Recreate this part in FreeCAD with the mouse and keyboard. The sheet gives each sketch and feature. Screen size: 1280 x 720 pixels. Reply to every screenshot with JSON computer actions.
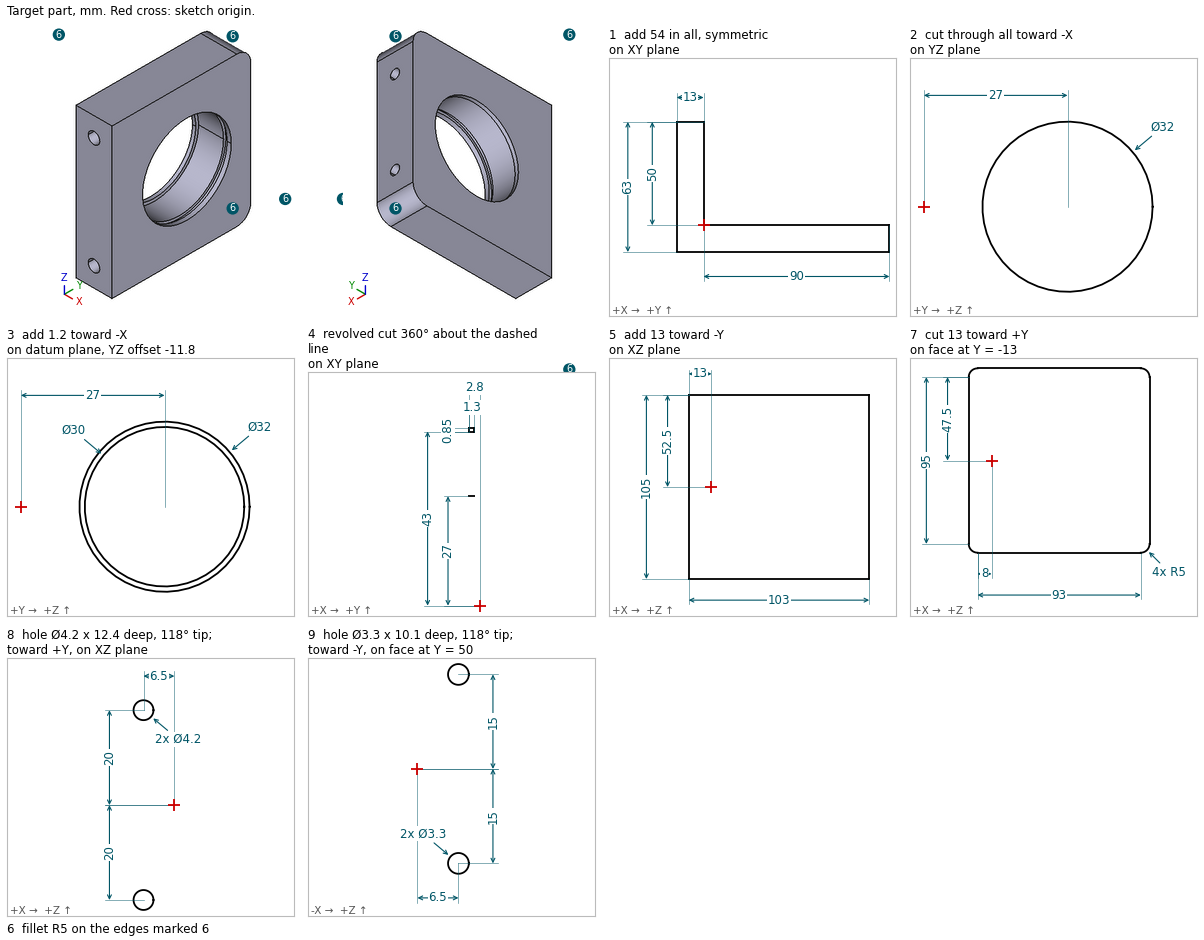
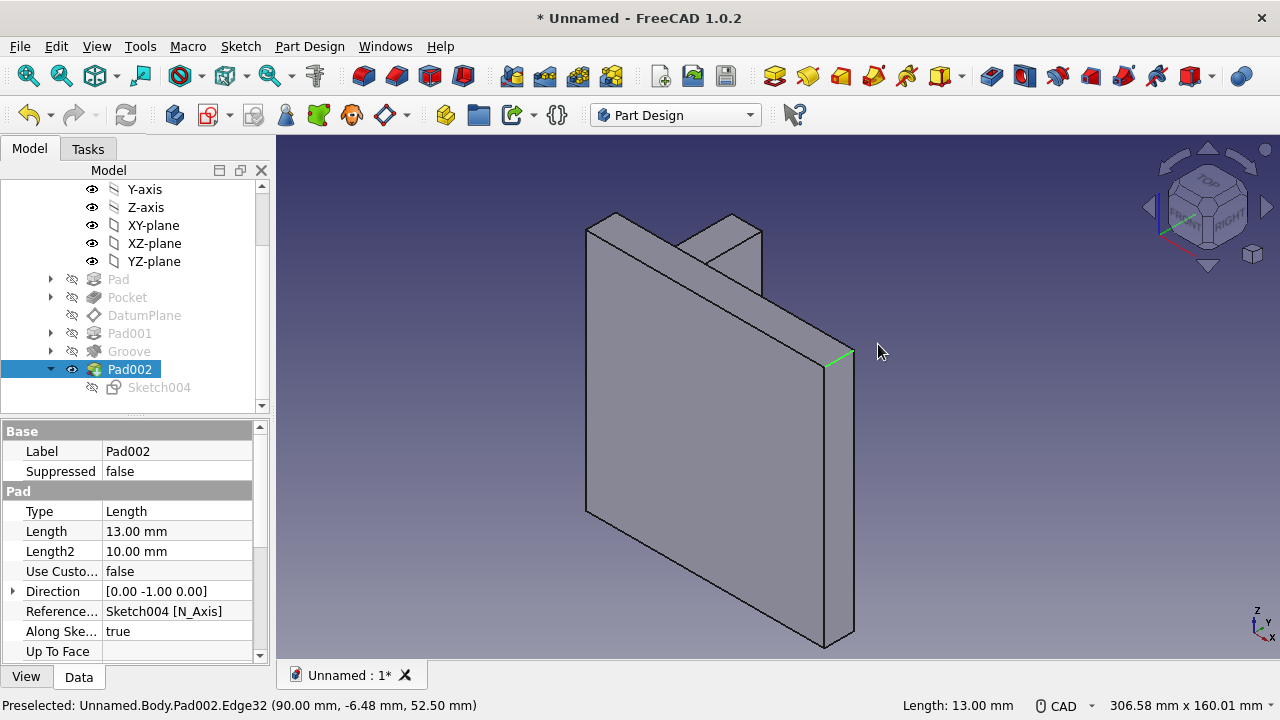
{"action": "key", "text": "2"}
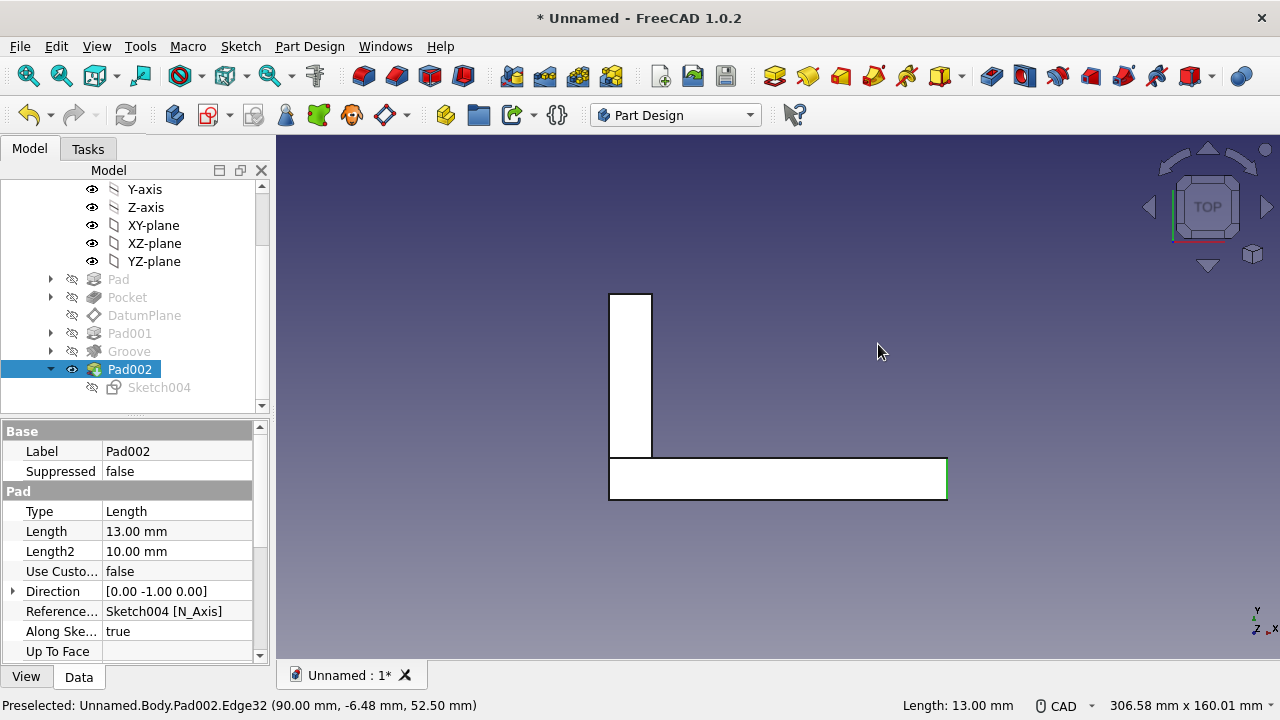
{"action": "left_click", "coordinate": [29, 76]}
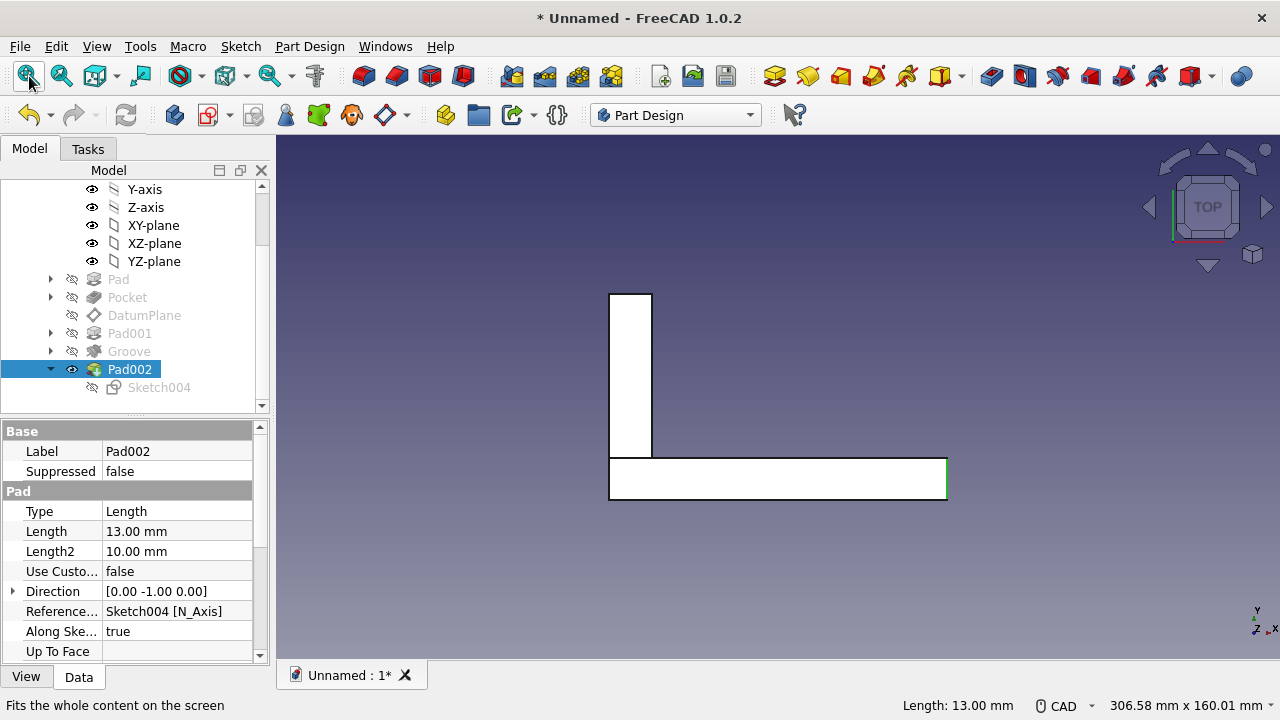
{"action": "left_click", "coordinate": [631, 293], "text": "ctrl"}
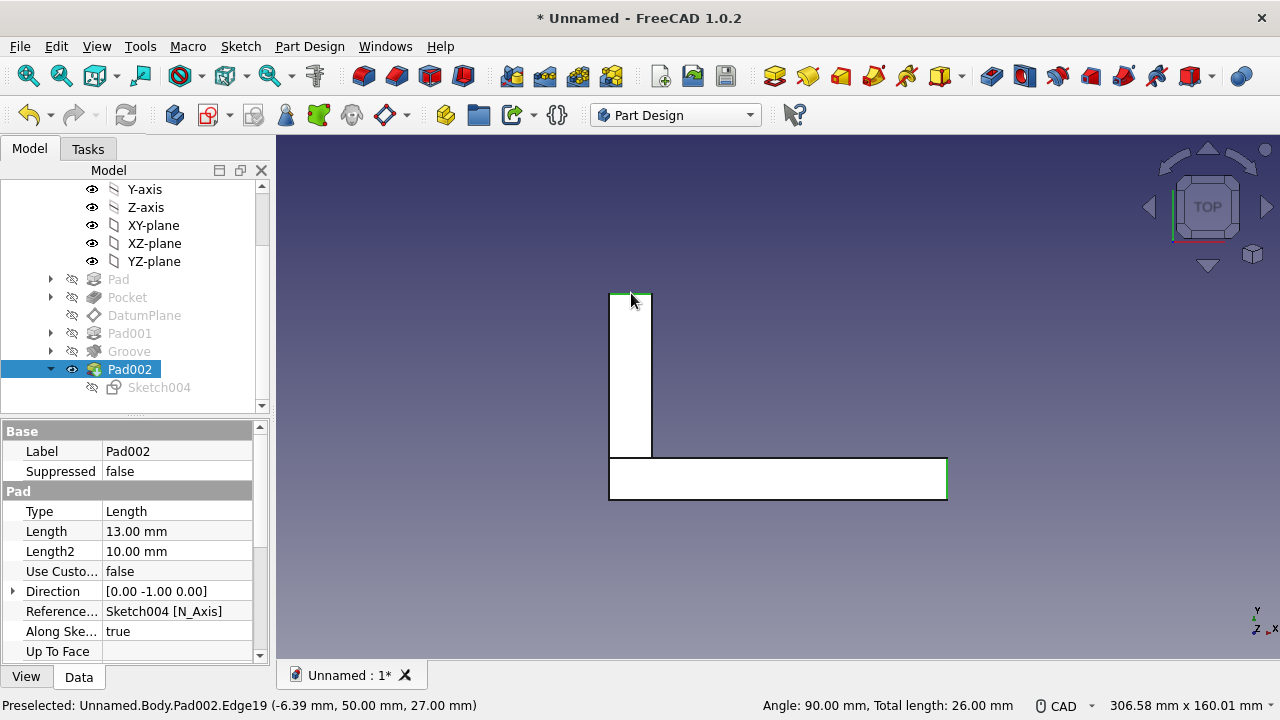
{"action": "left_click", "coordinate": [609, 478], "text": "ctrl"}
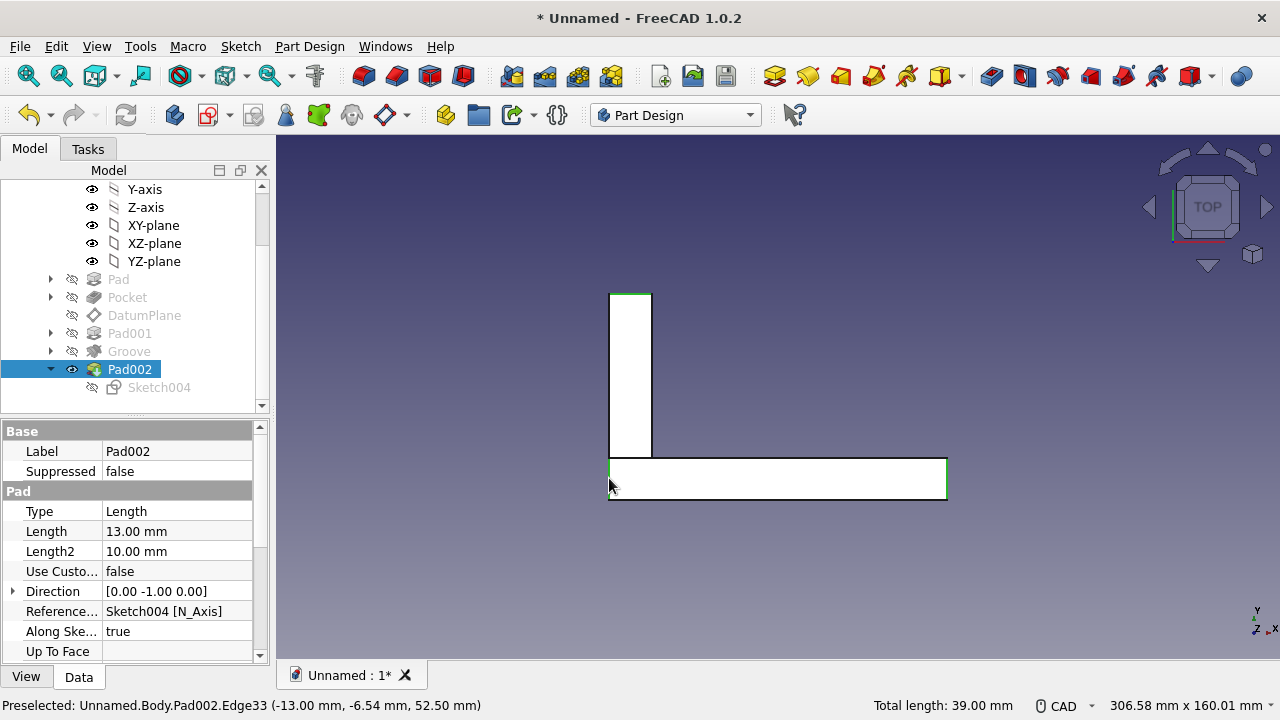
{"action": "key", "text": "1"}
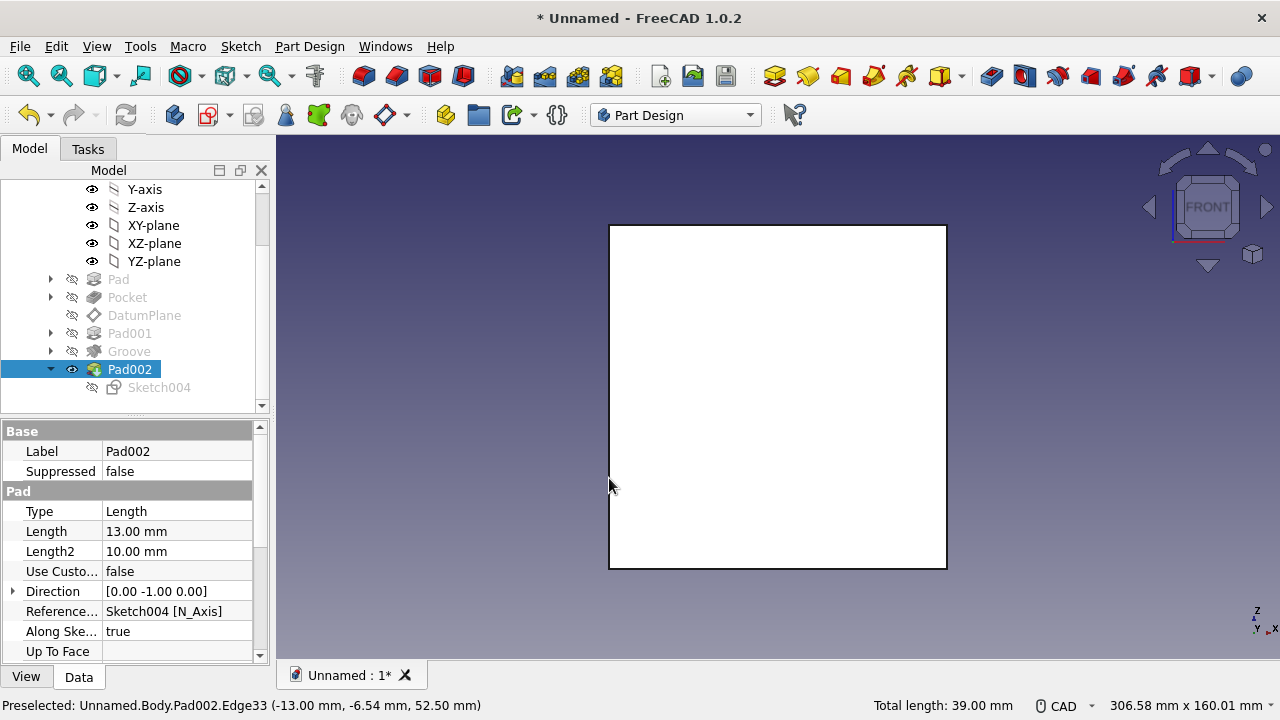
{"action": "key", "text": "3"}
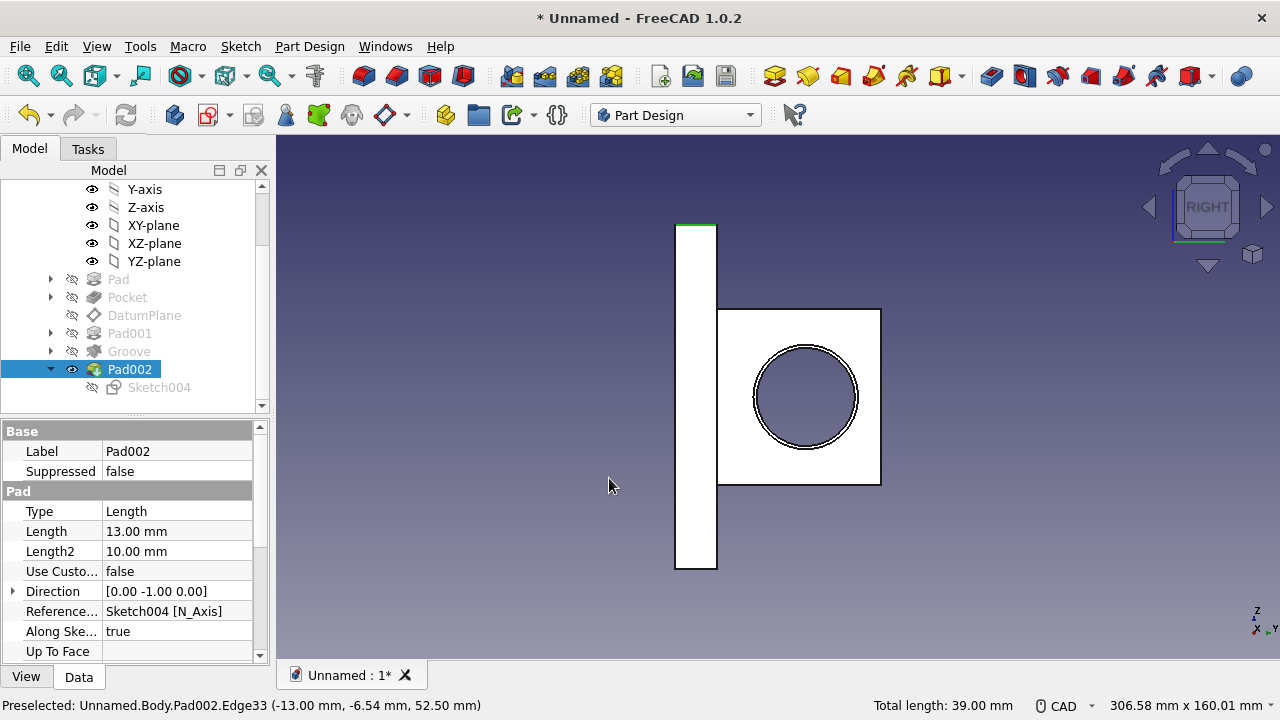
{"action": "left_click", "coordinate": [696, 568], "text": "ctrl"}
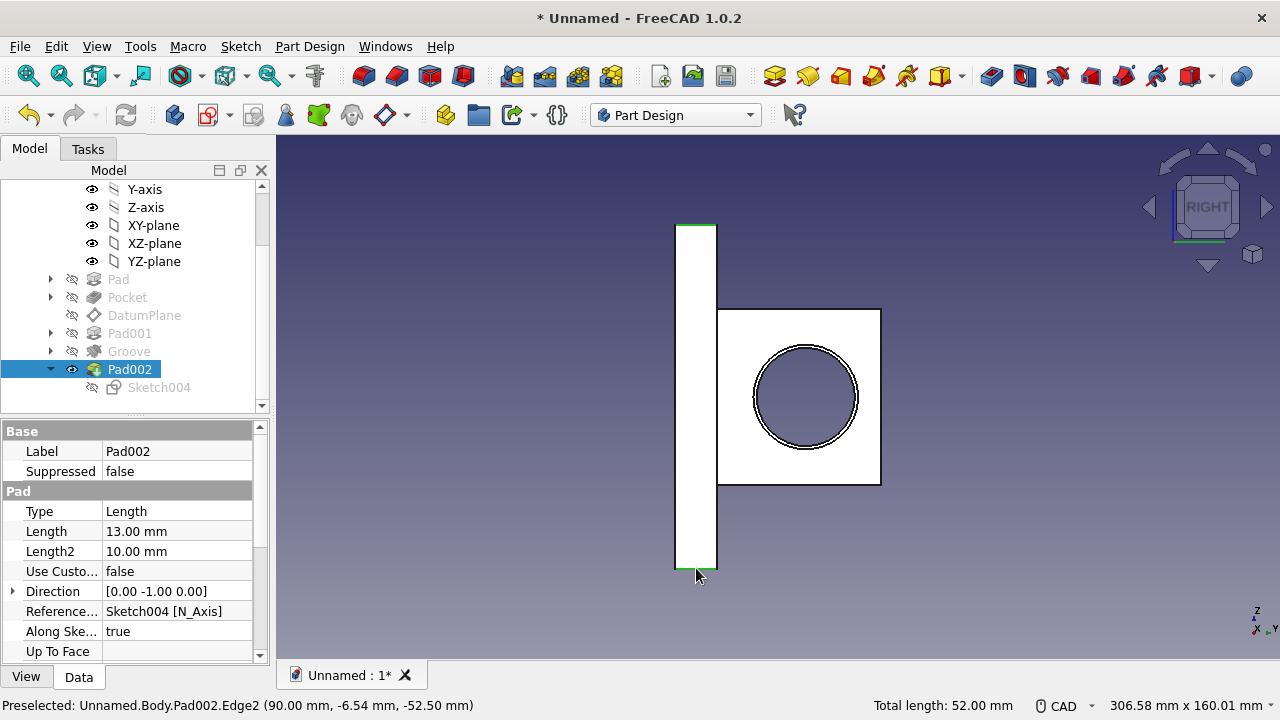
{"action": "key", "text": "5"}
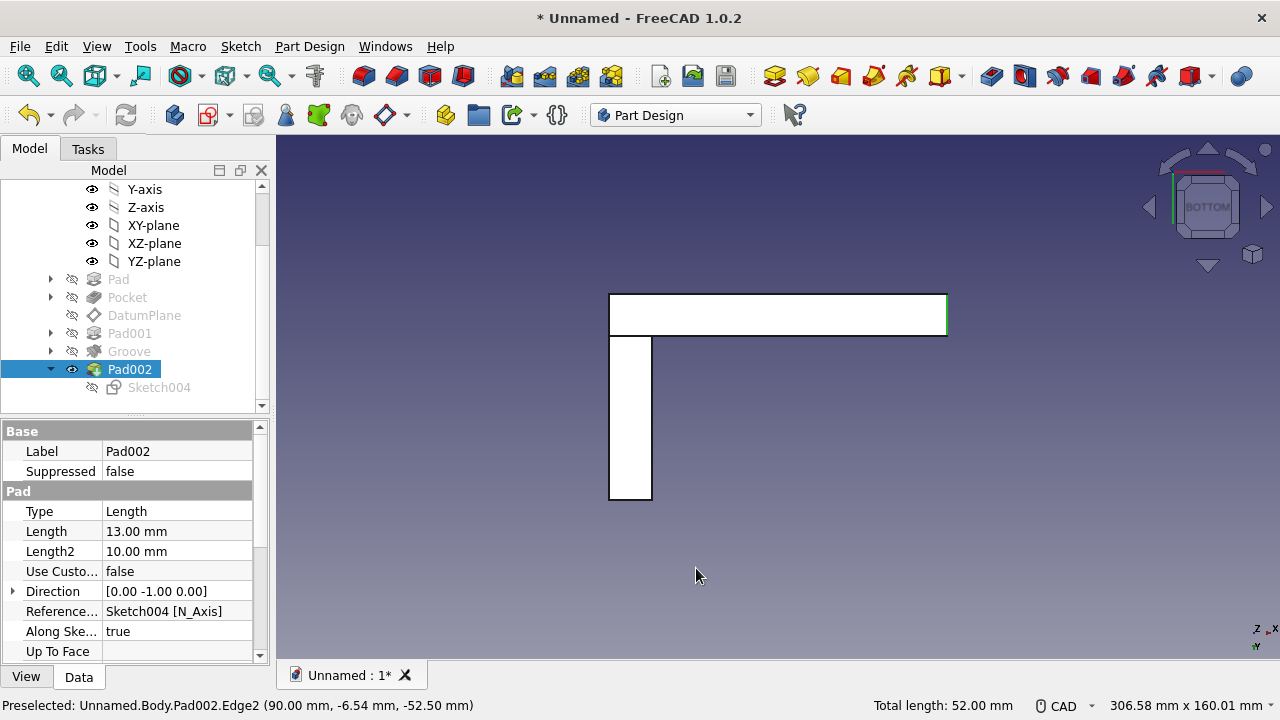
{"action": "left_click", "coordinate": [29, 76]}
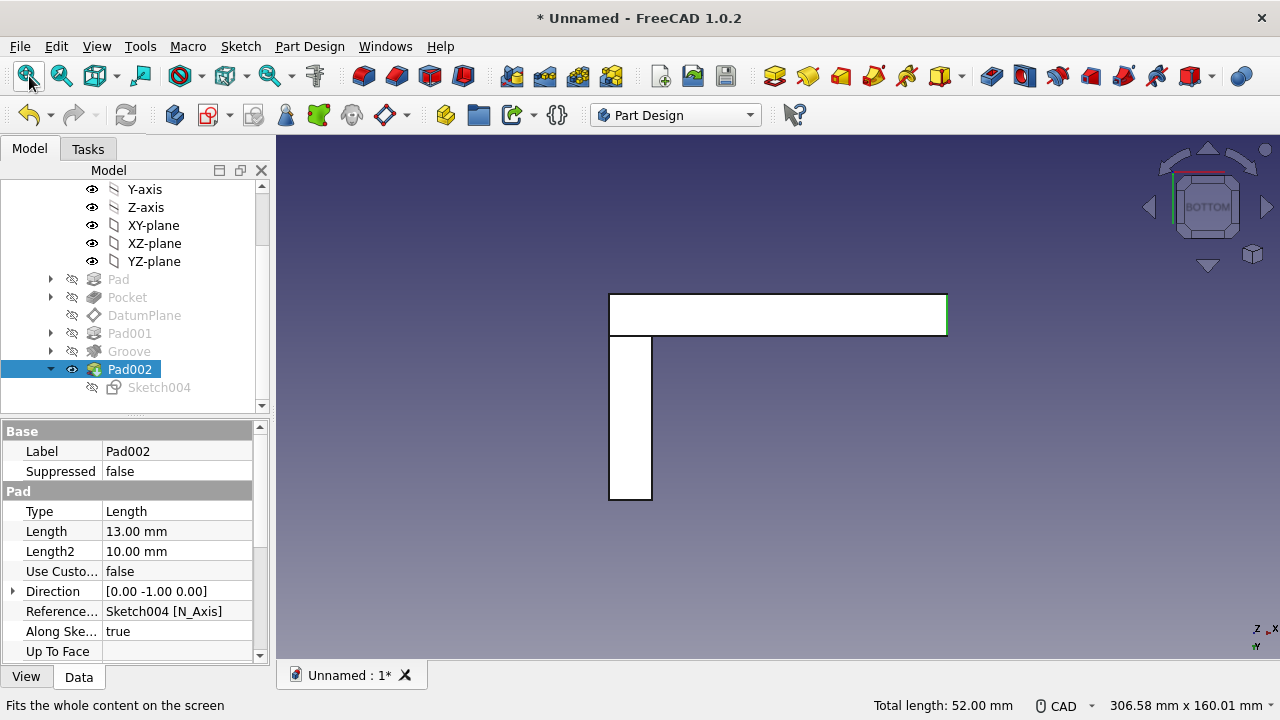
{"action": "left_click", "coordinate": [609, 314], "text": "ctrl"}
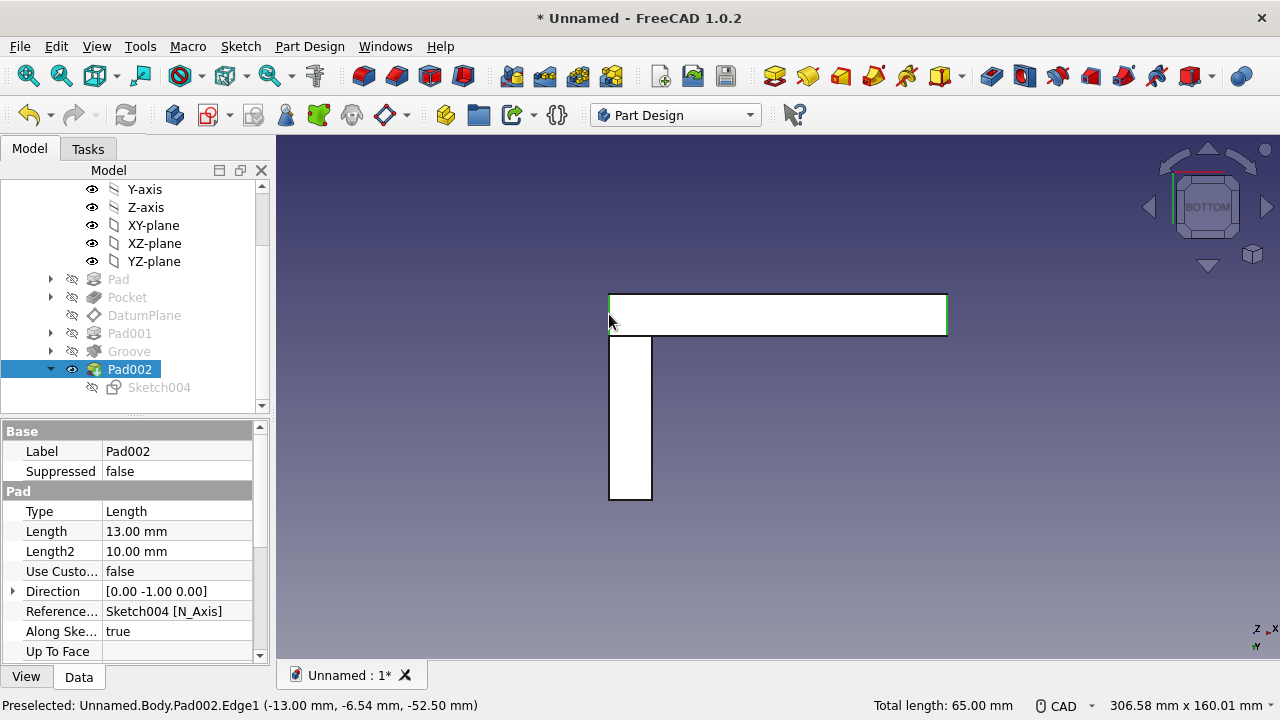
{"action": "left_click", "coordinate": [631, 499], "text": "ctrl"}